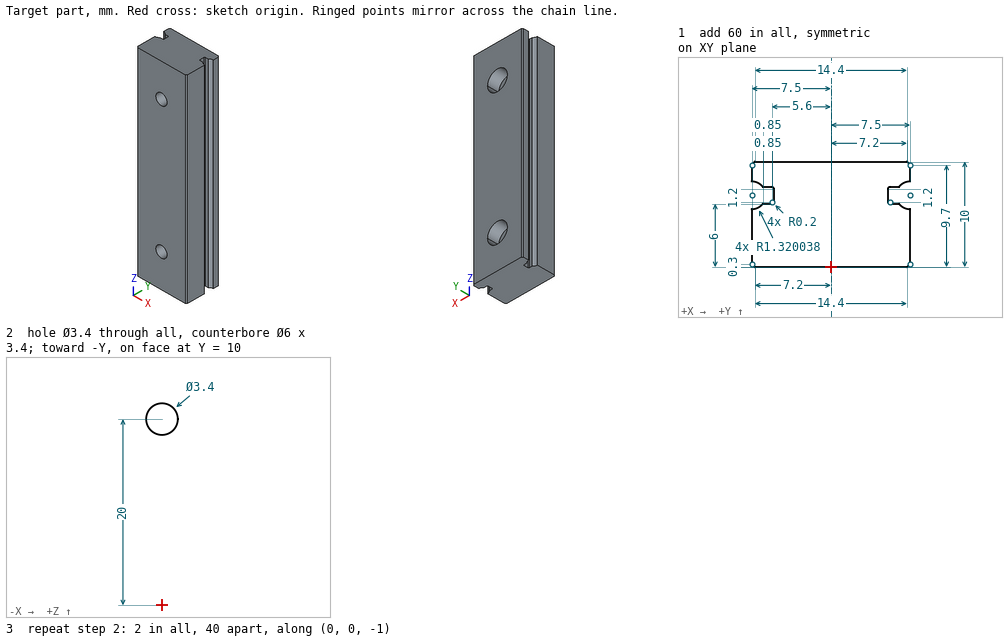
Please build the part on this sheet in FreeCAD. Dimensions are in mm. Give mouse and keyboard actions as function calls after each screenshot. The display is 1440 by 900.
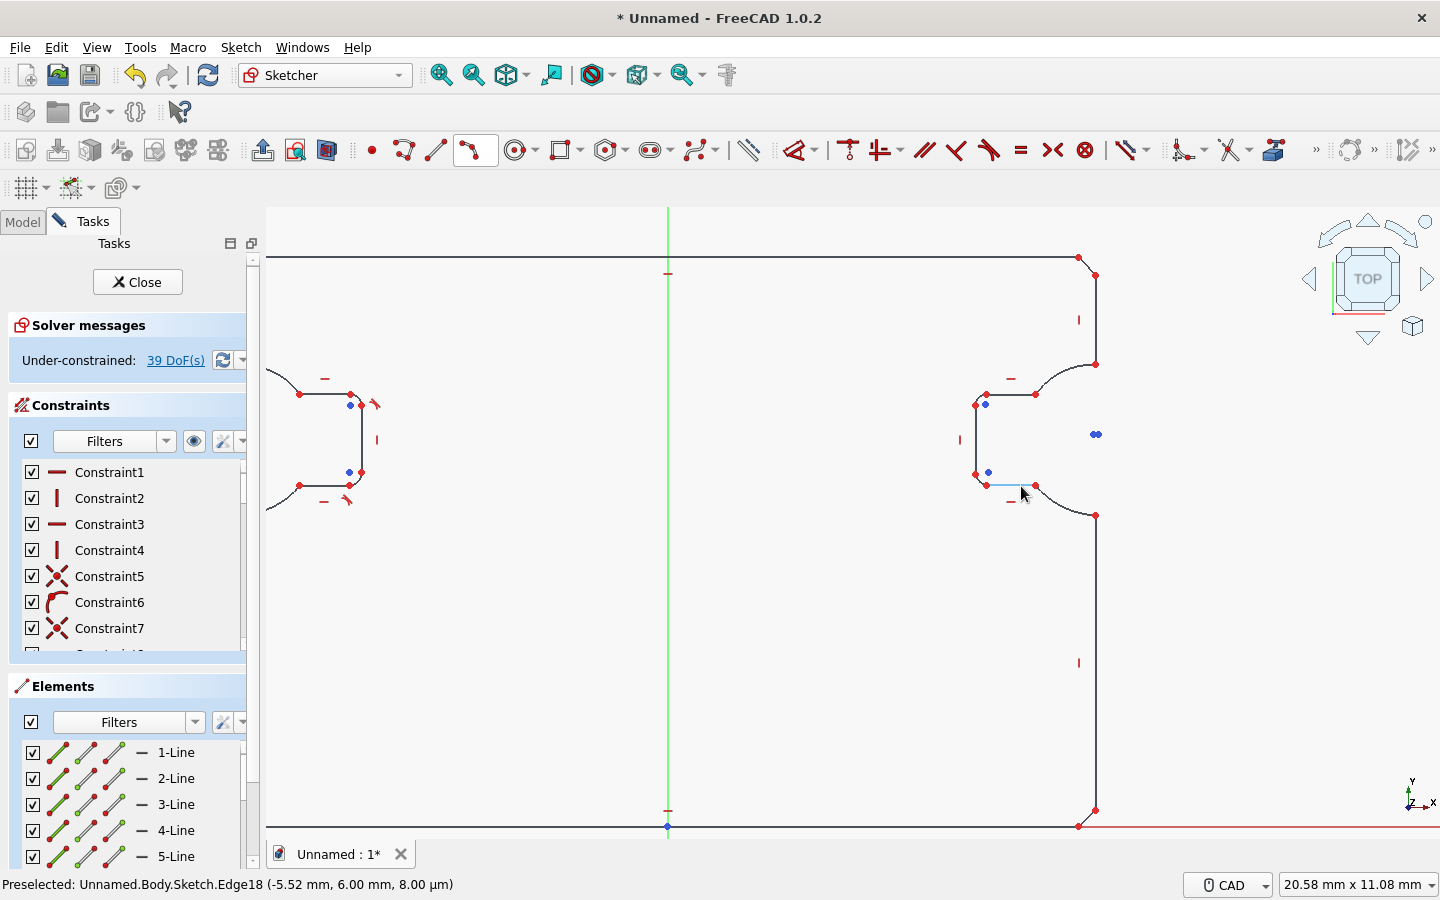
click(1021, 485)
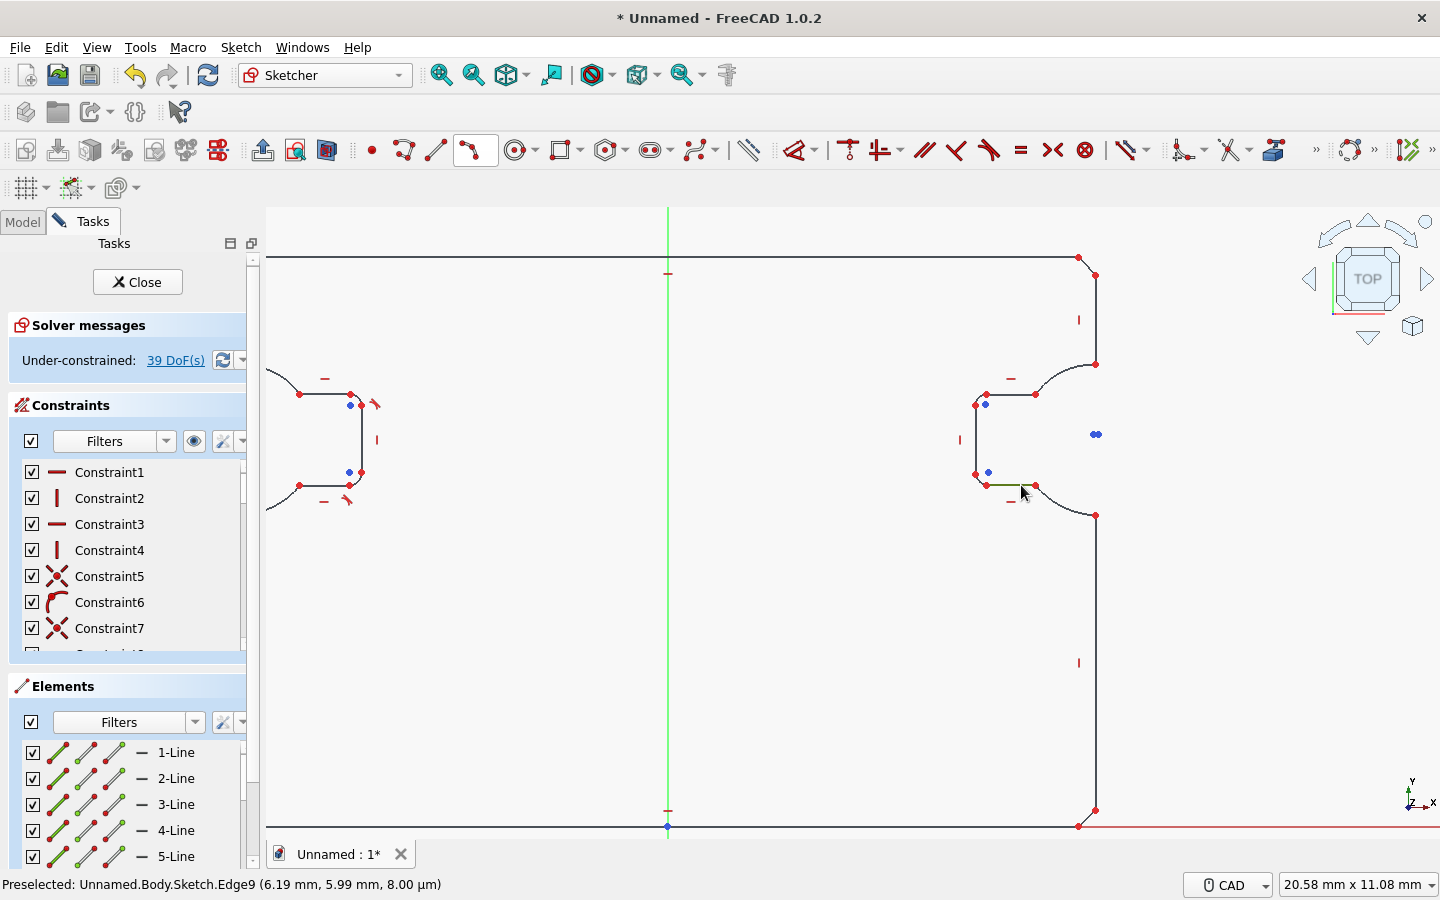
scroll(980, 482, up, 3)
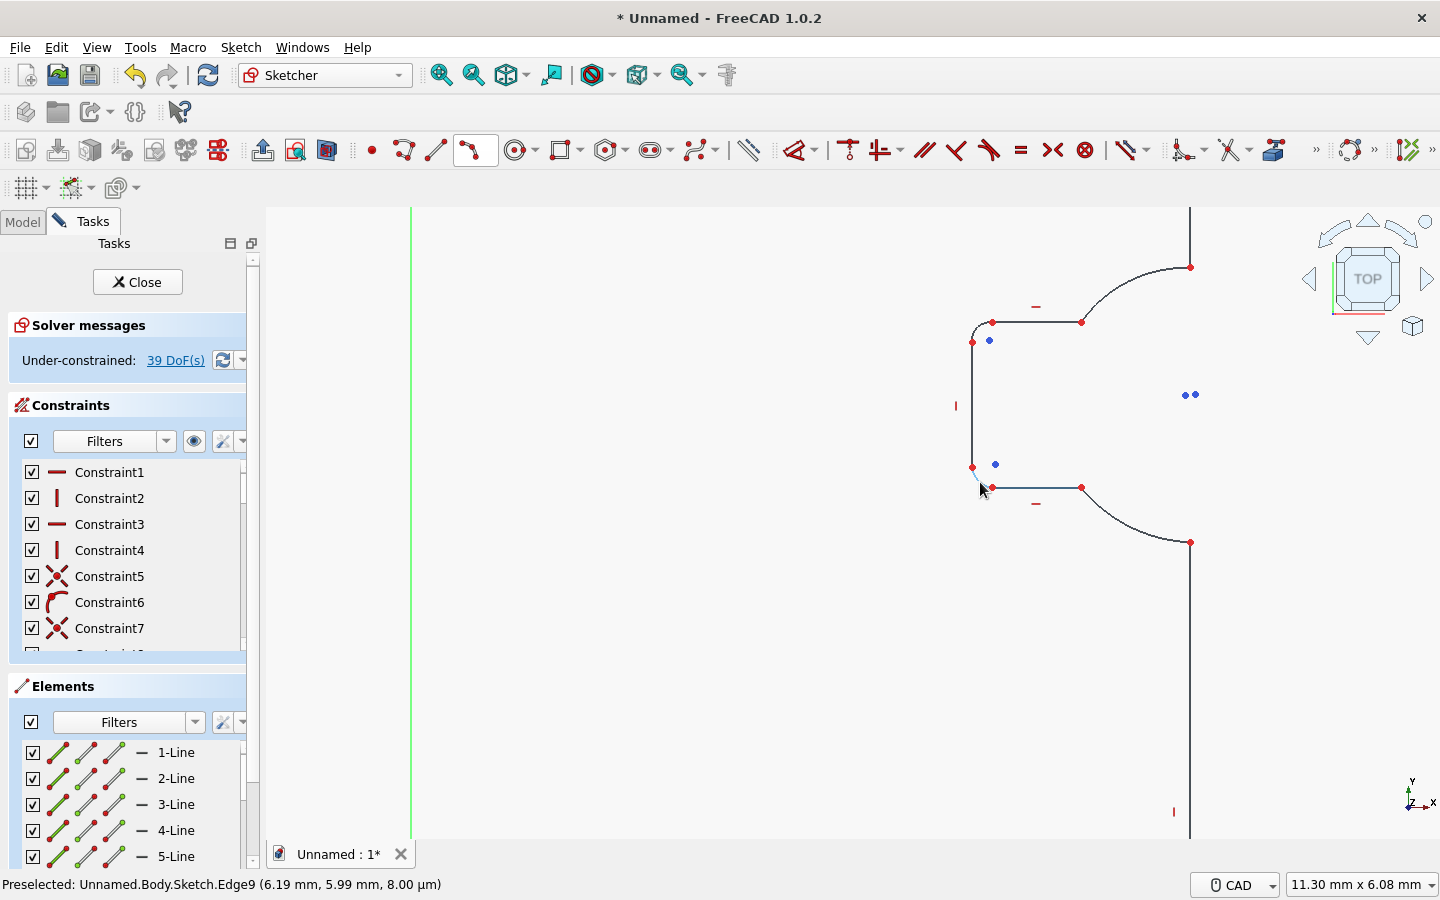
click(979, 481)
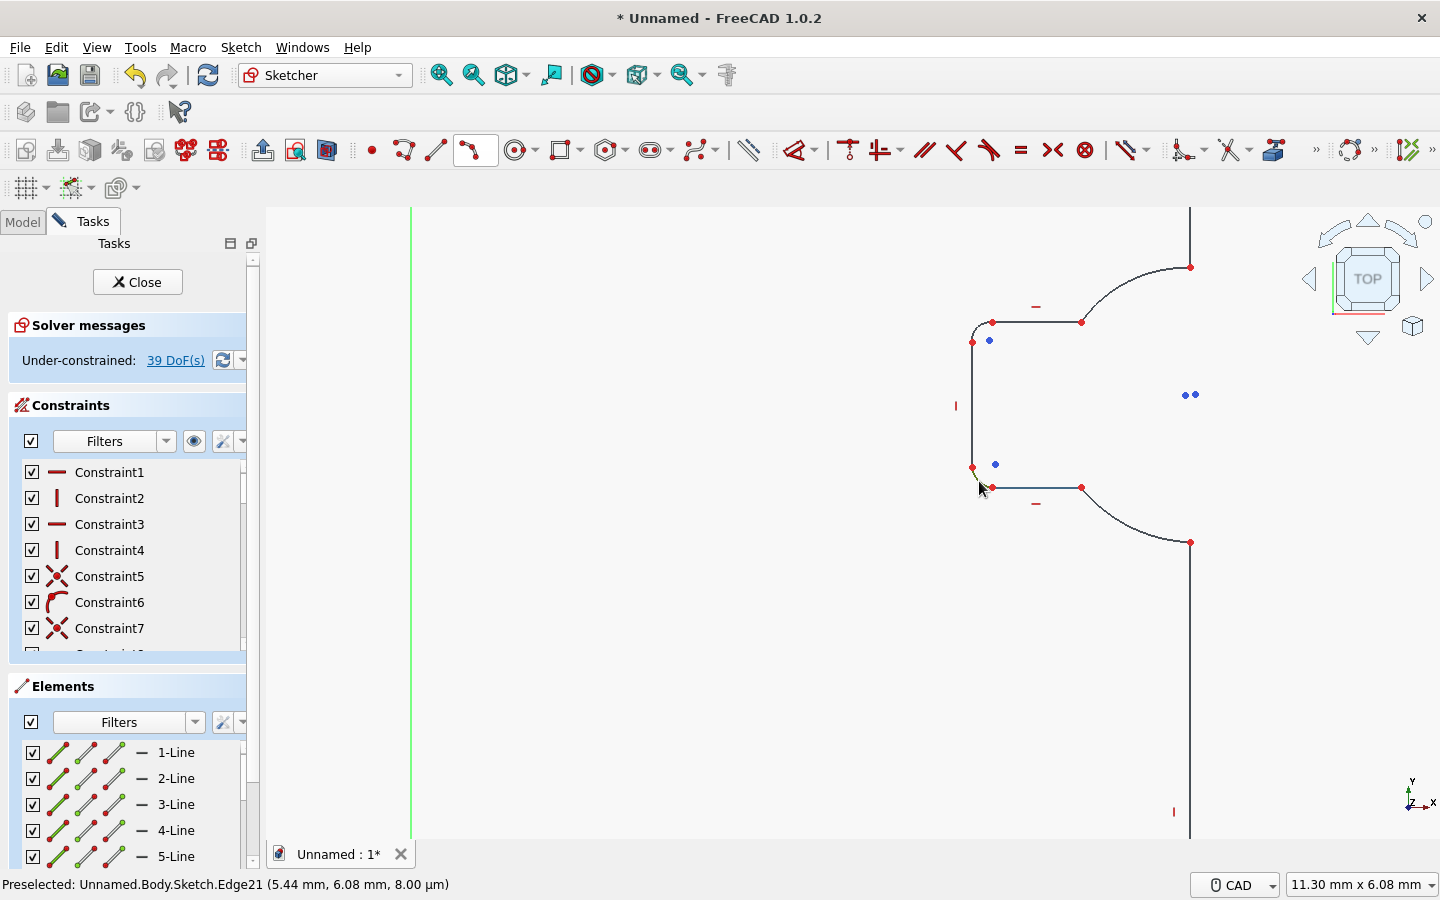
key(t)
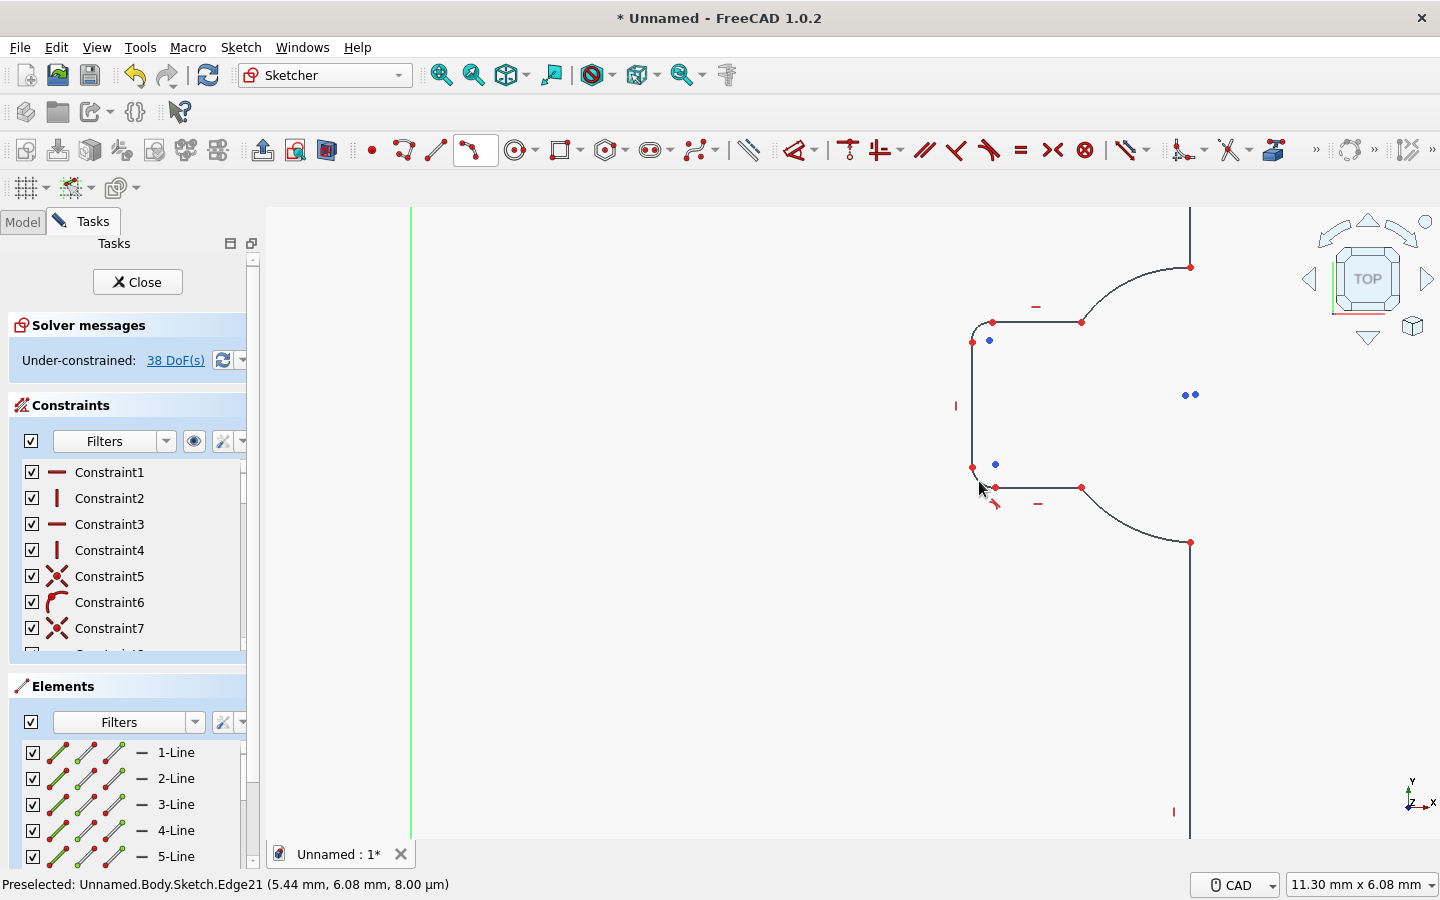
click(972, 430)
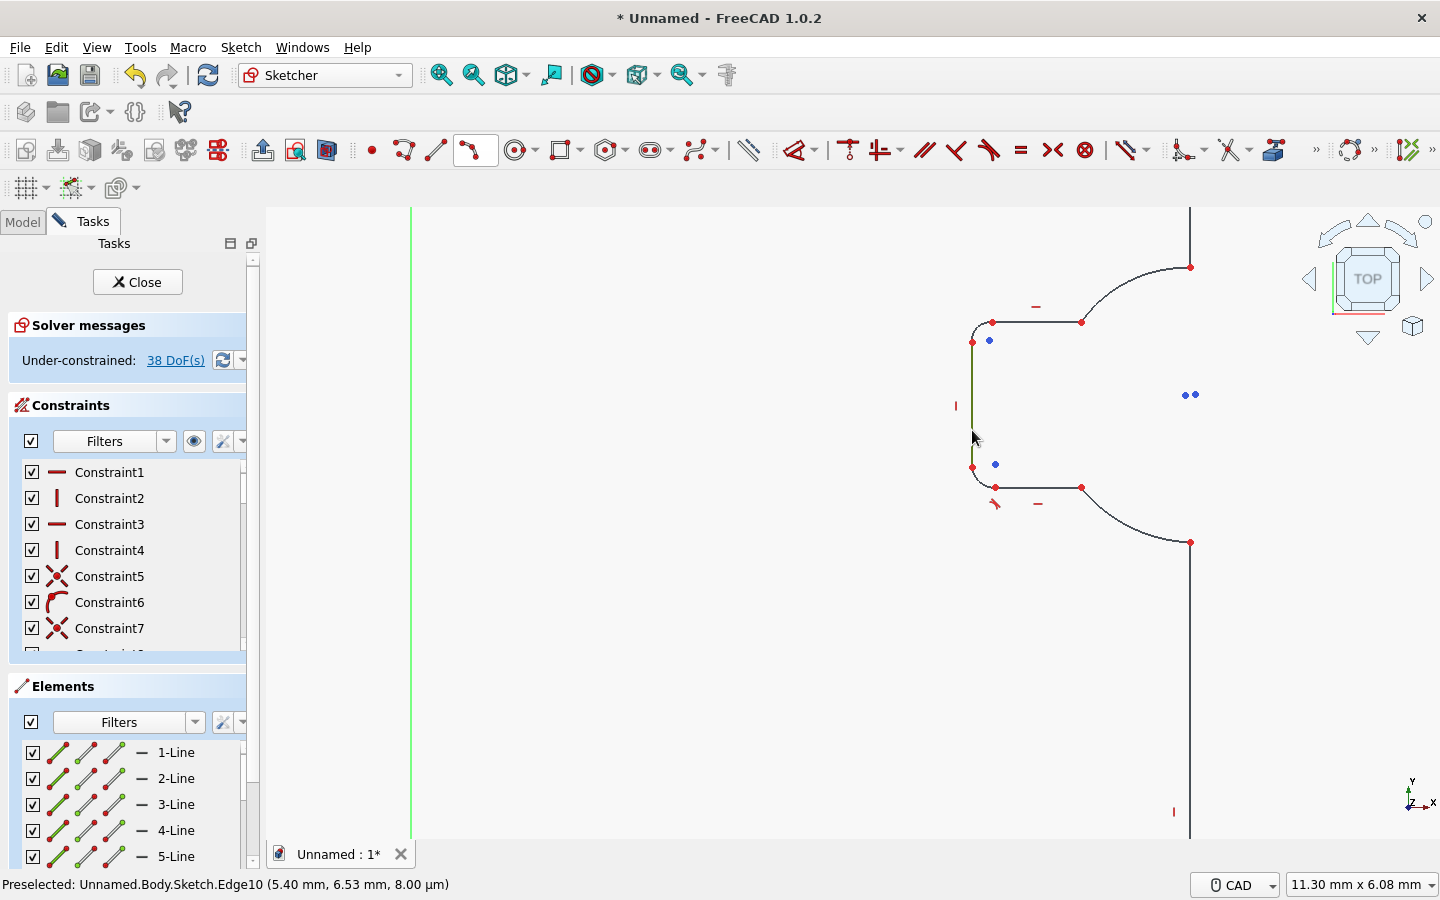
scroll(976, 477, up, 2)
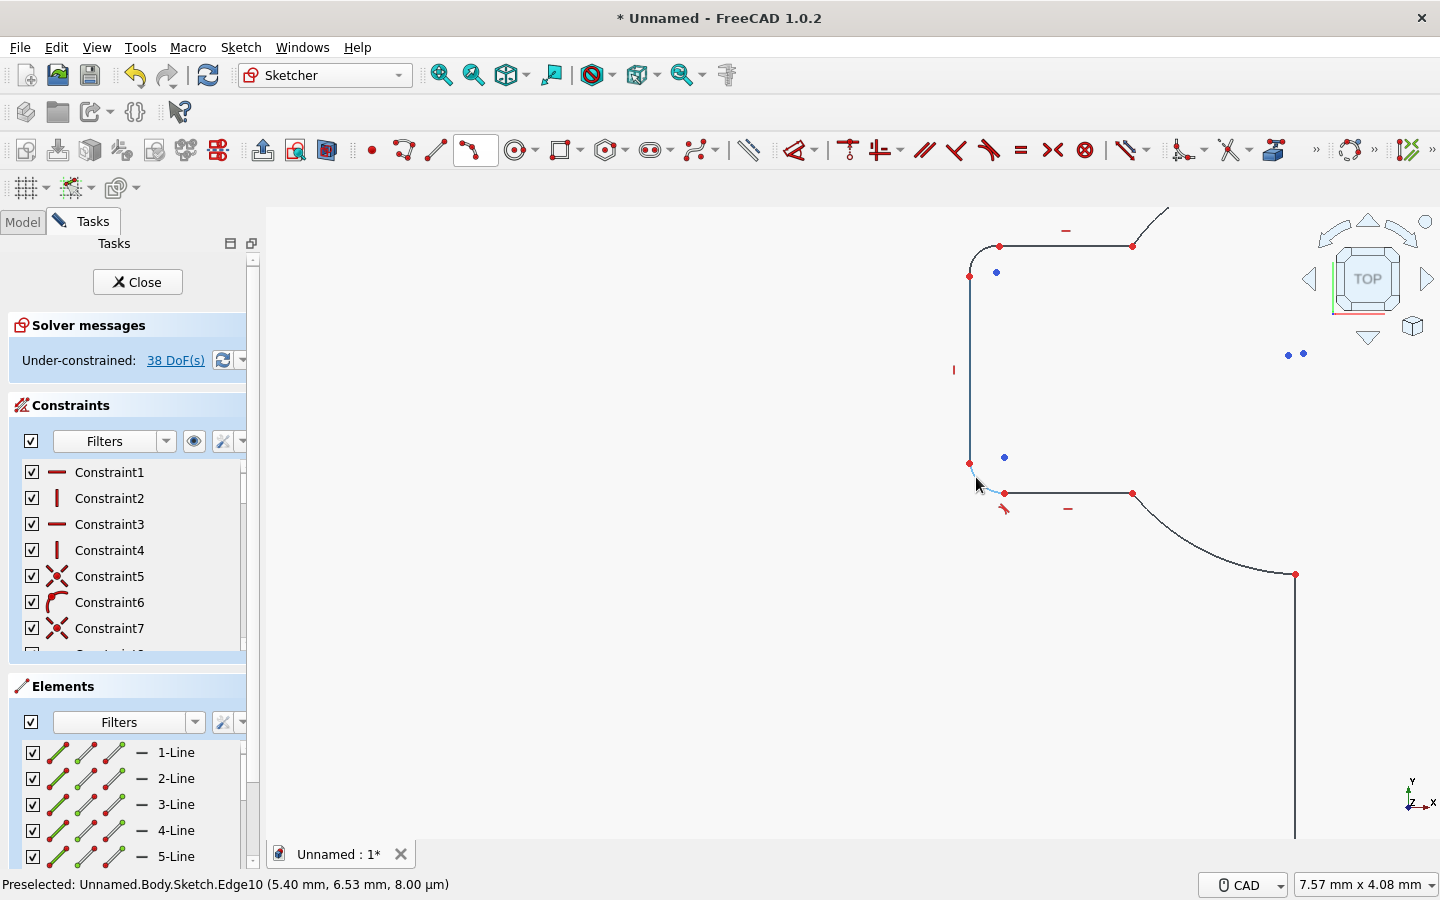
click(975, 477)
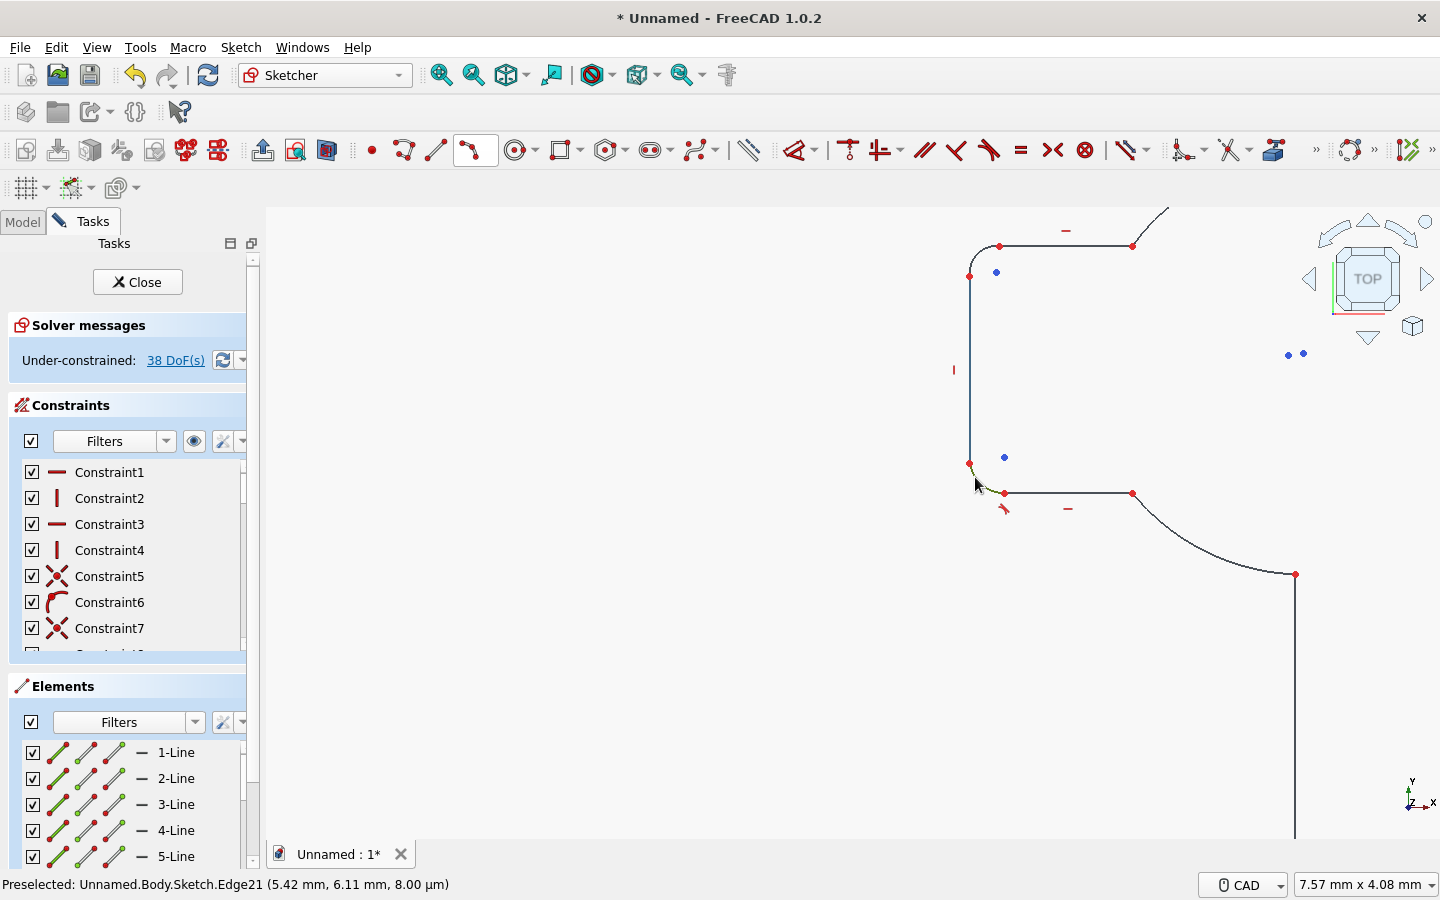
click(990, 150)